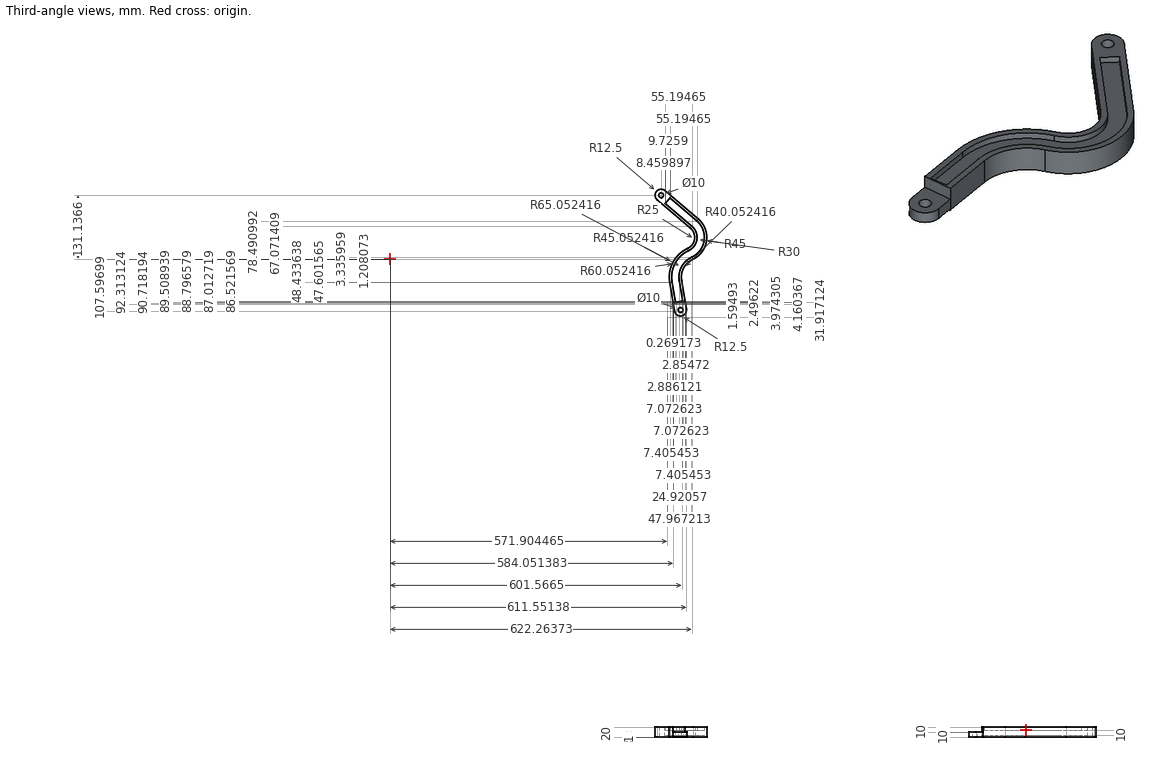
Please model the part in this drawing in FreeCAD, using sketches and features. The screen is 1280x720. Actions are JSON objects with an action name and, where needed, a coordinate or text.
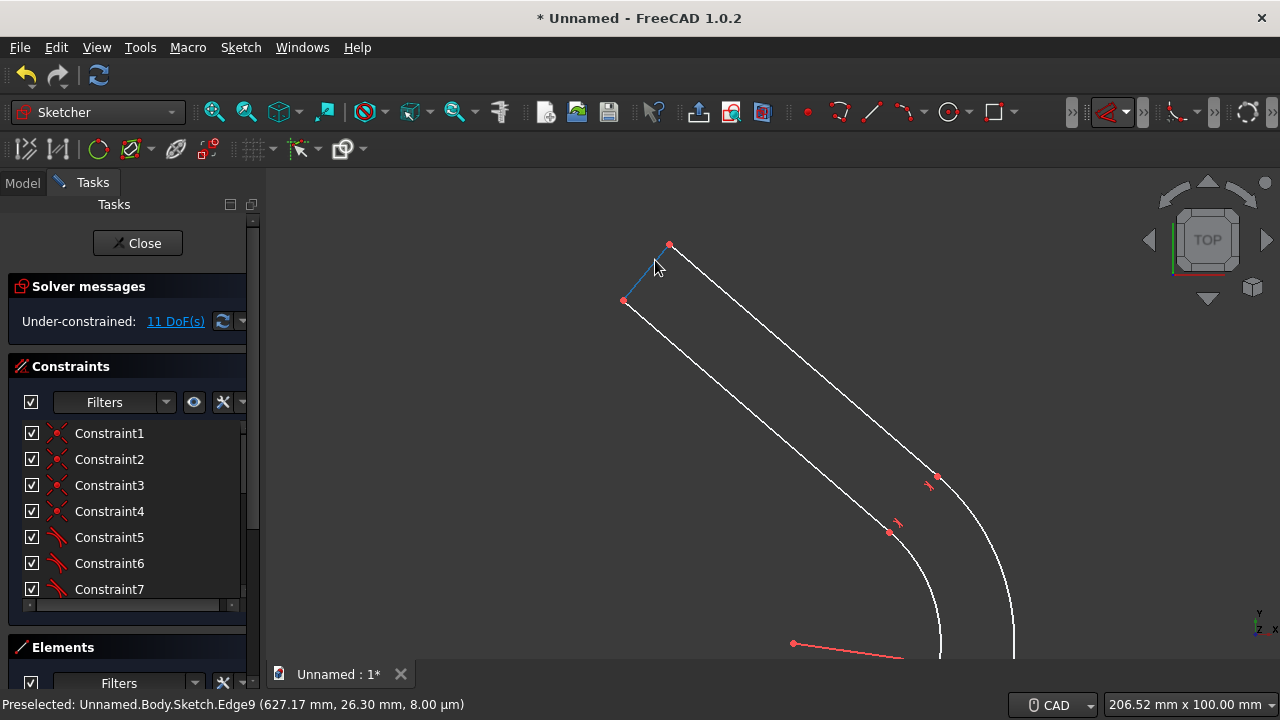
{"action": "left_click", "coordinate": [656, 261]}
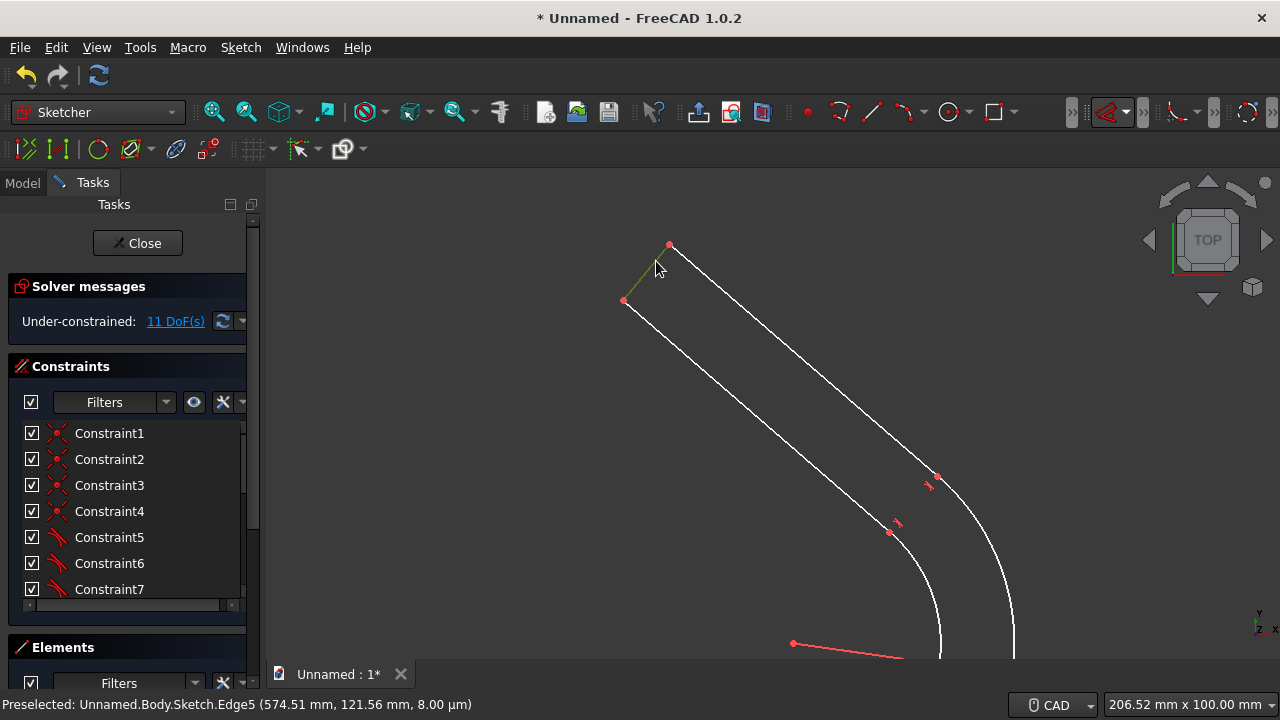
{"action": "key", "text": "l"}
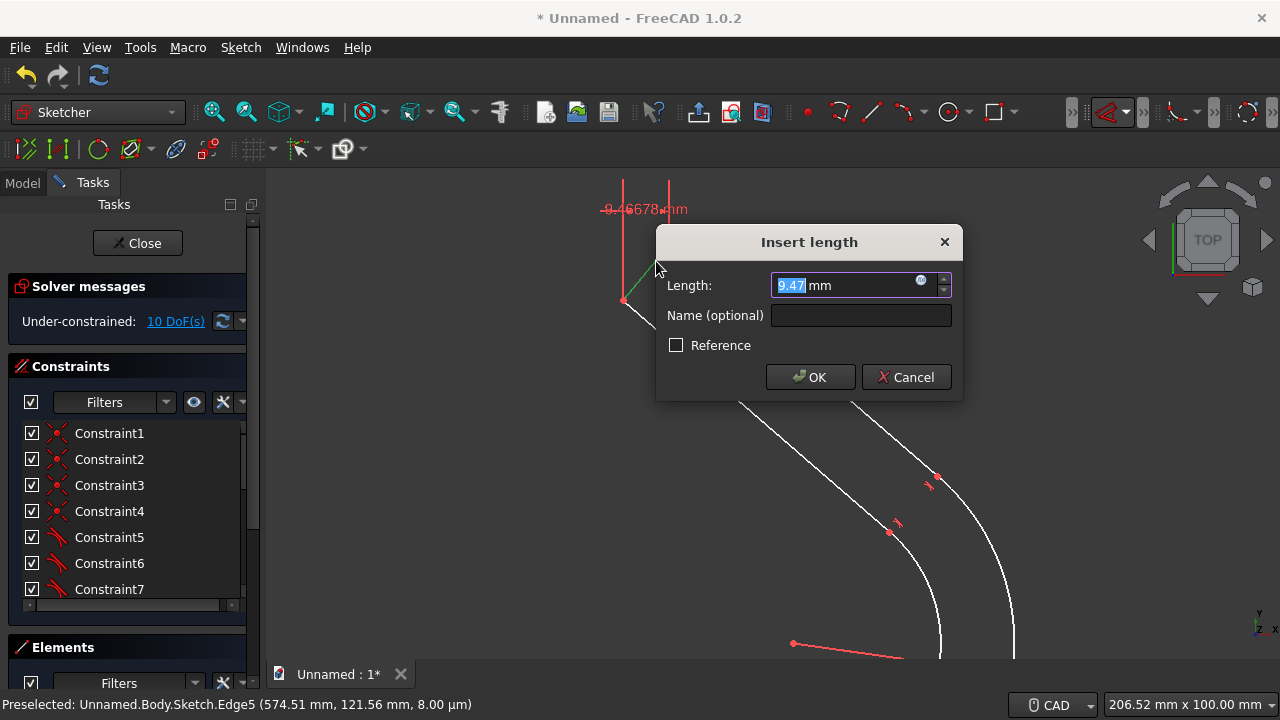
{"action": "type", "text": "9.7259"}
{"action": "key", "text": "Return"}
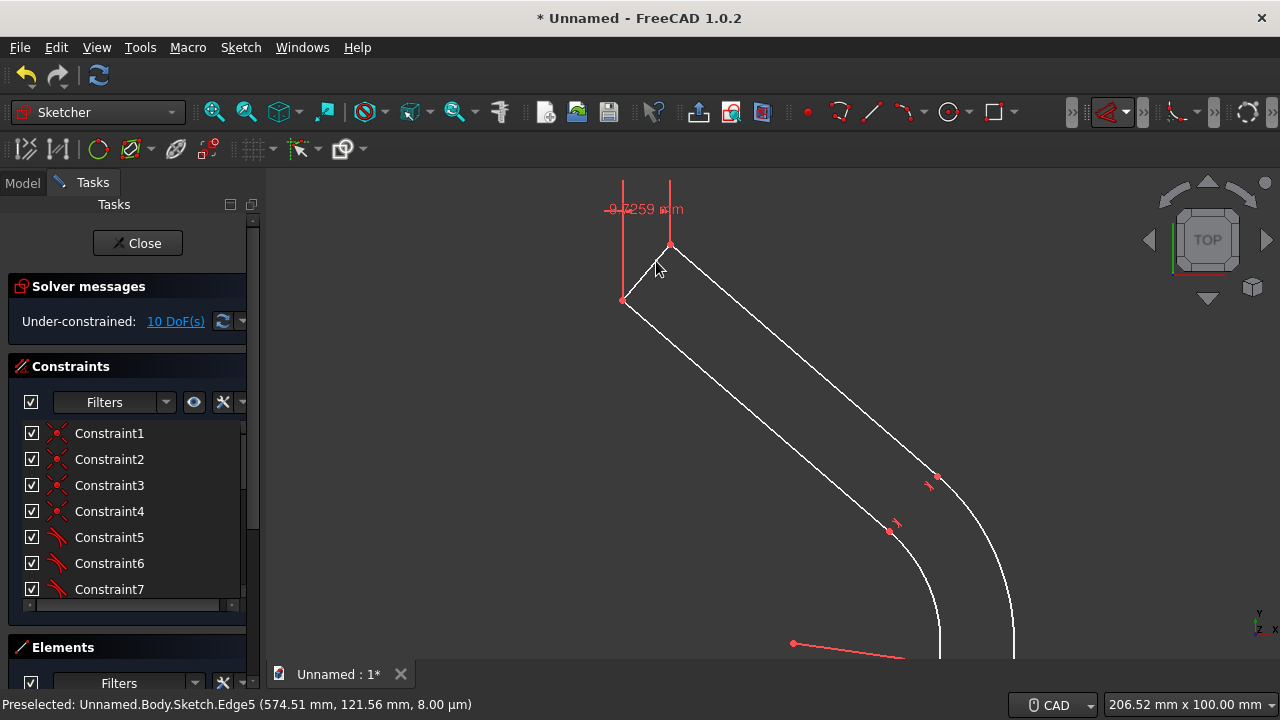
{"action": "scroll", "coordinate": [655, 260], "scroll_direction": "down", "scroll_amount": 6}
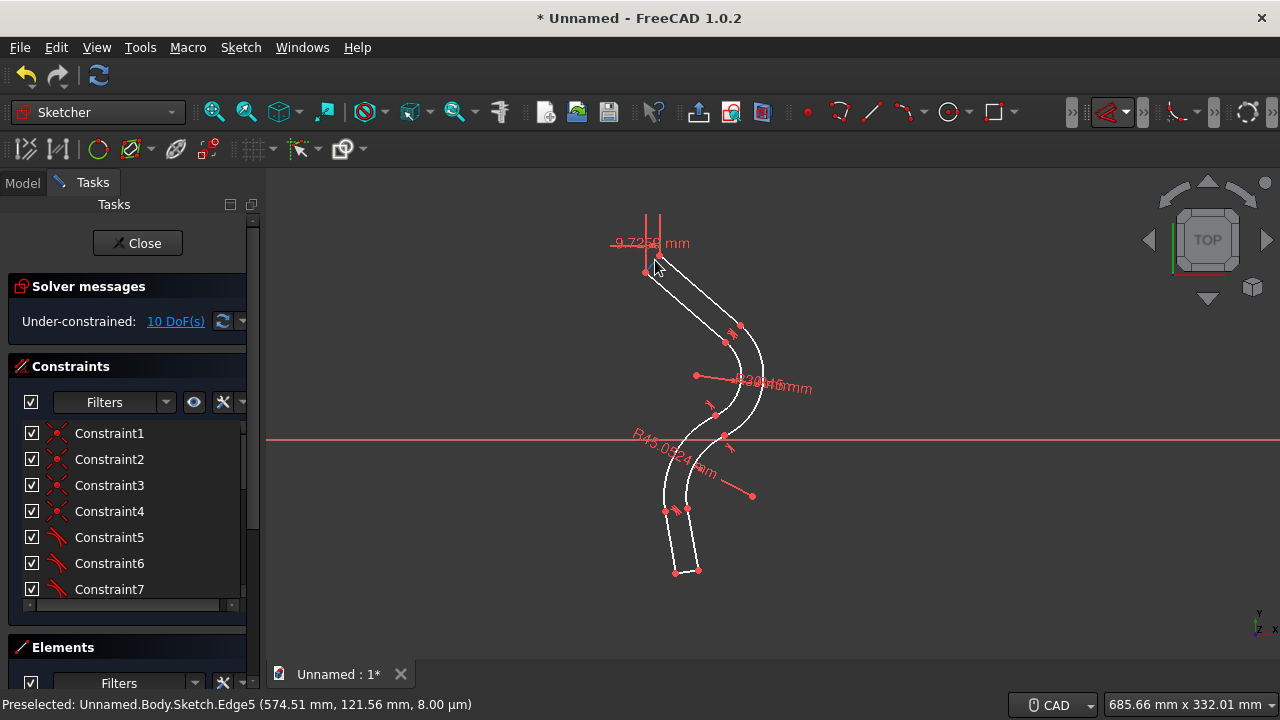
{"action": "scroll", "coordinate": [683, 572], "scroll_direction": "up", "scroll_amount": 12}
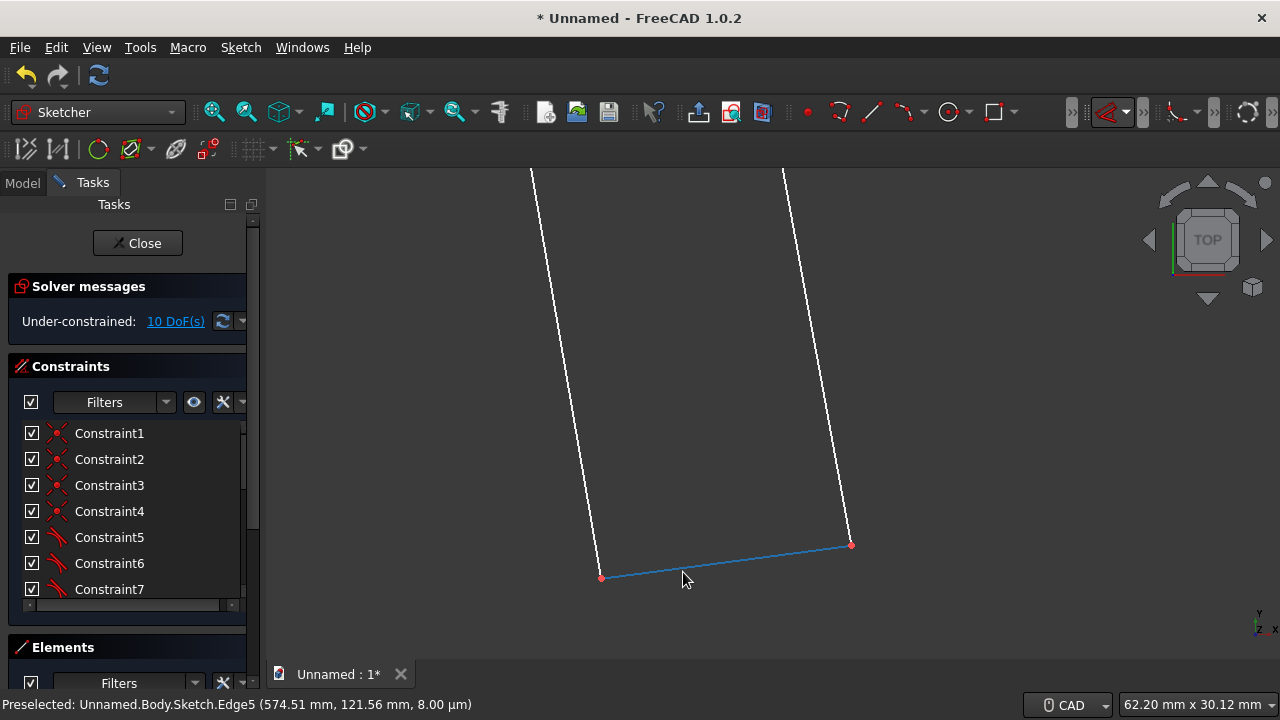
{"action": "left_click", "coordinate": [676, 569]}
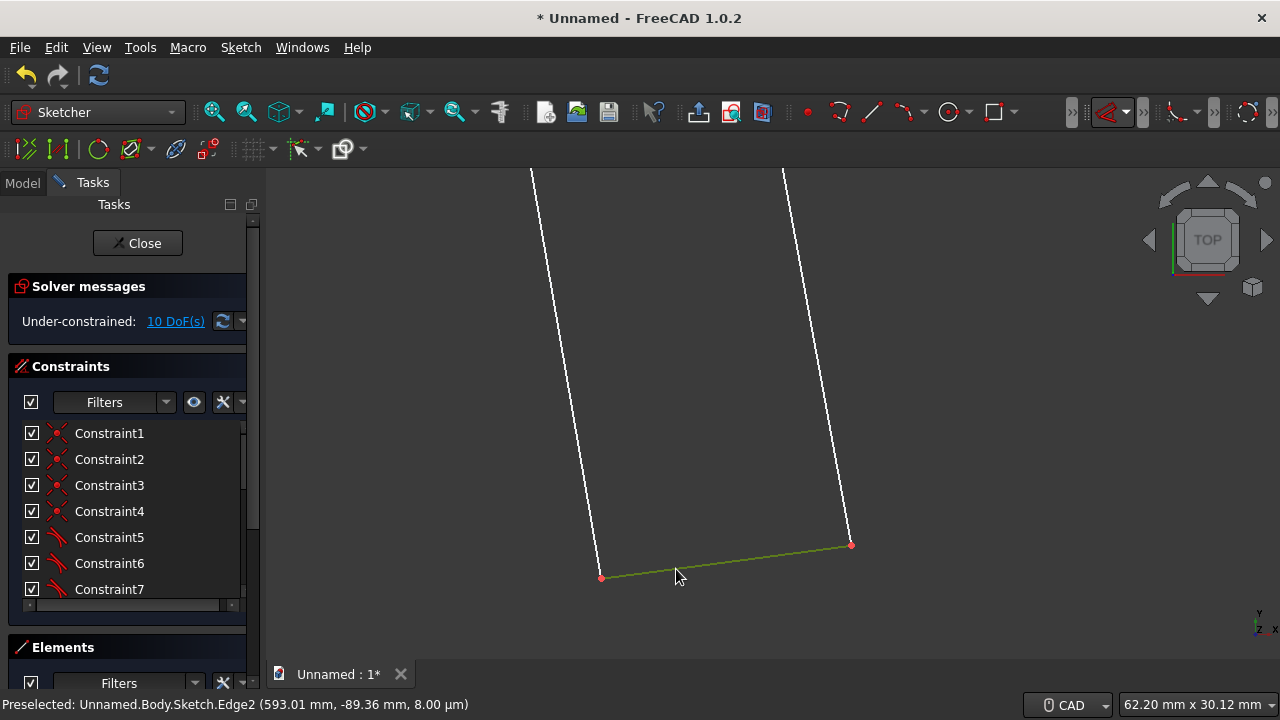
{"action": "key", "text": "i"}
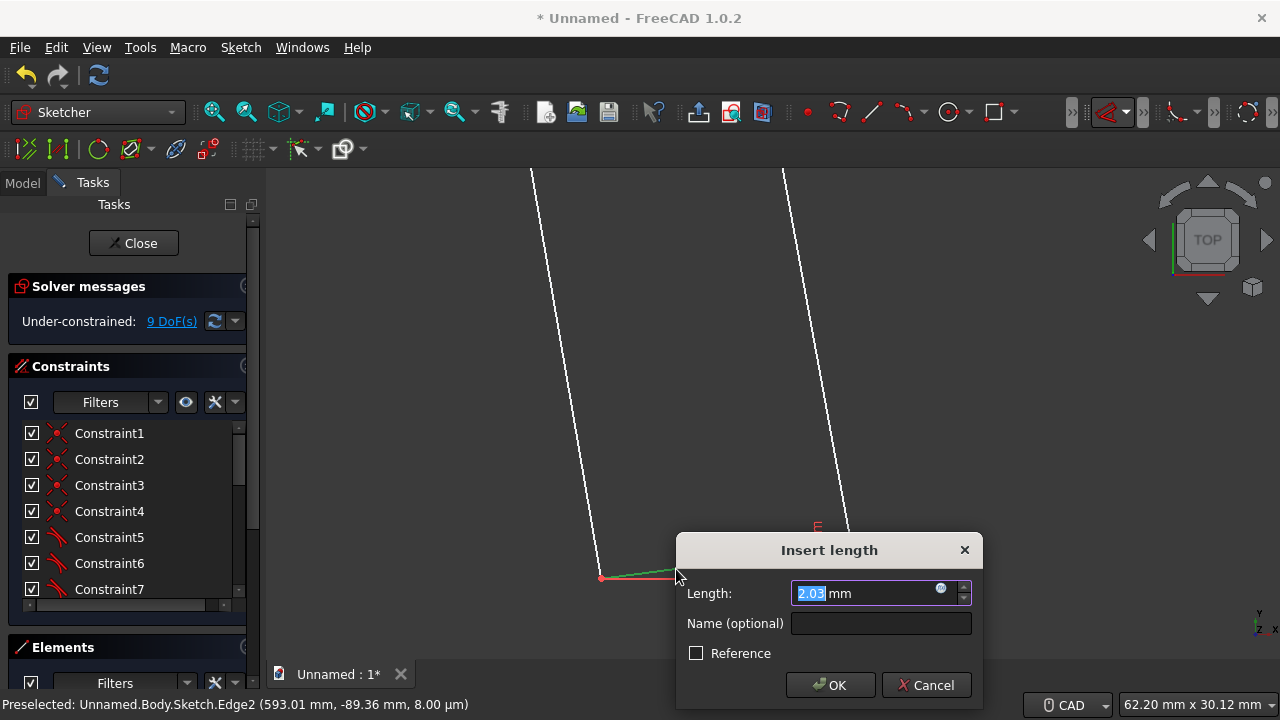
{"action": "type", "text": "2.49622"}
{"action": "key", "text": "Return"}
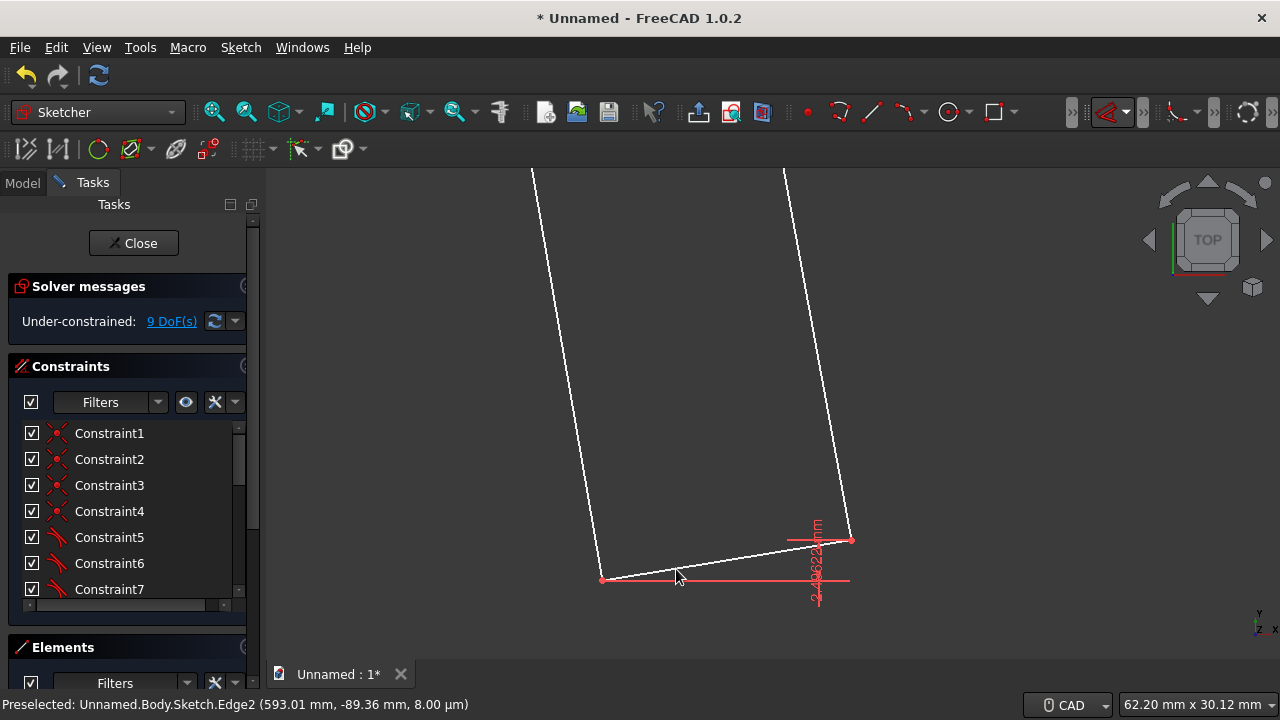
{"action": "scroll", "coordinate": [683, 573], "scroll_direction": "down", "scroll_amount": 12}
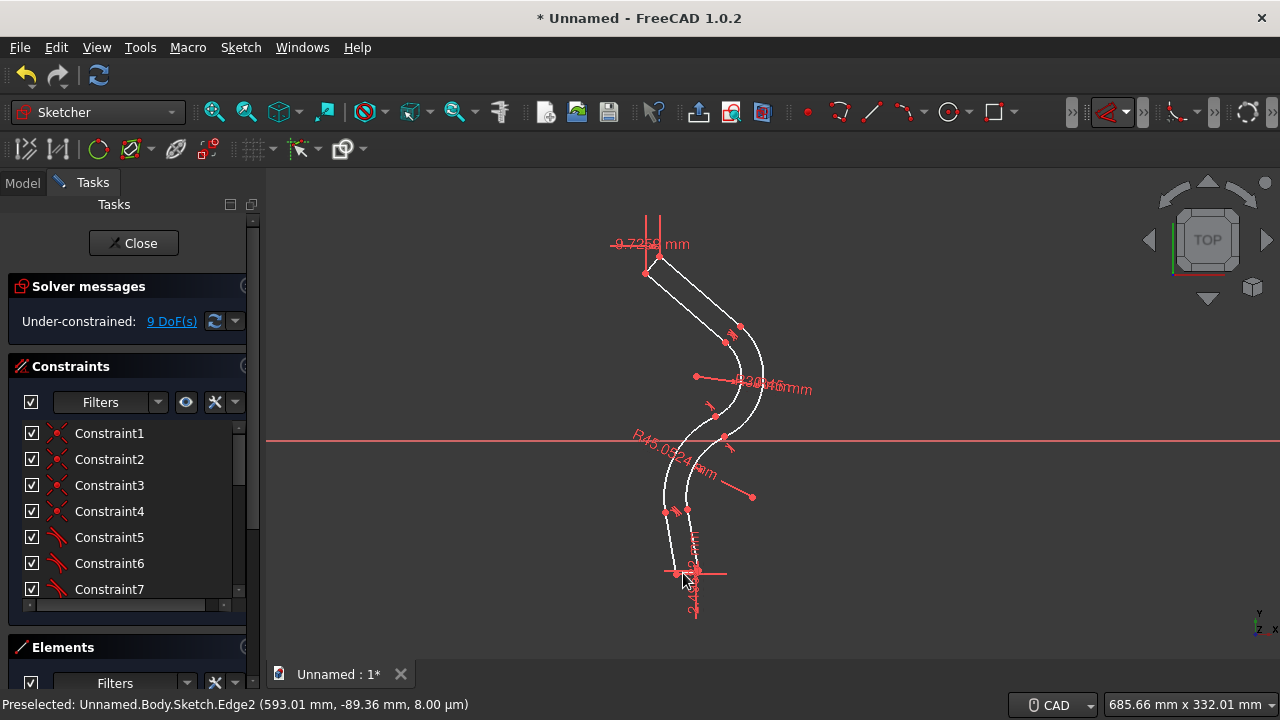
{"action": "scroll", "coordinate": [725, 437], "scroll_direction": "up", "scroll_amount": 11}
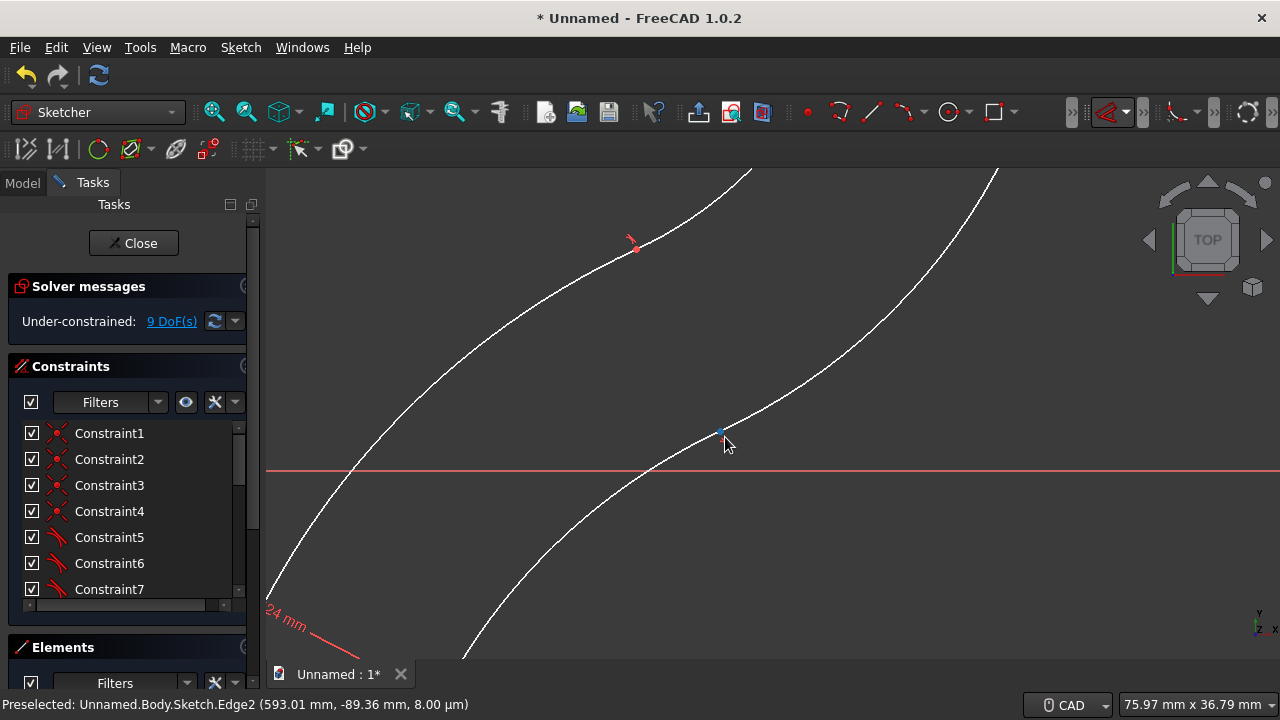
{"action": "left_click", "coordinate": [720, 431]}